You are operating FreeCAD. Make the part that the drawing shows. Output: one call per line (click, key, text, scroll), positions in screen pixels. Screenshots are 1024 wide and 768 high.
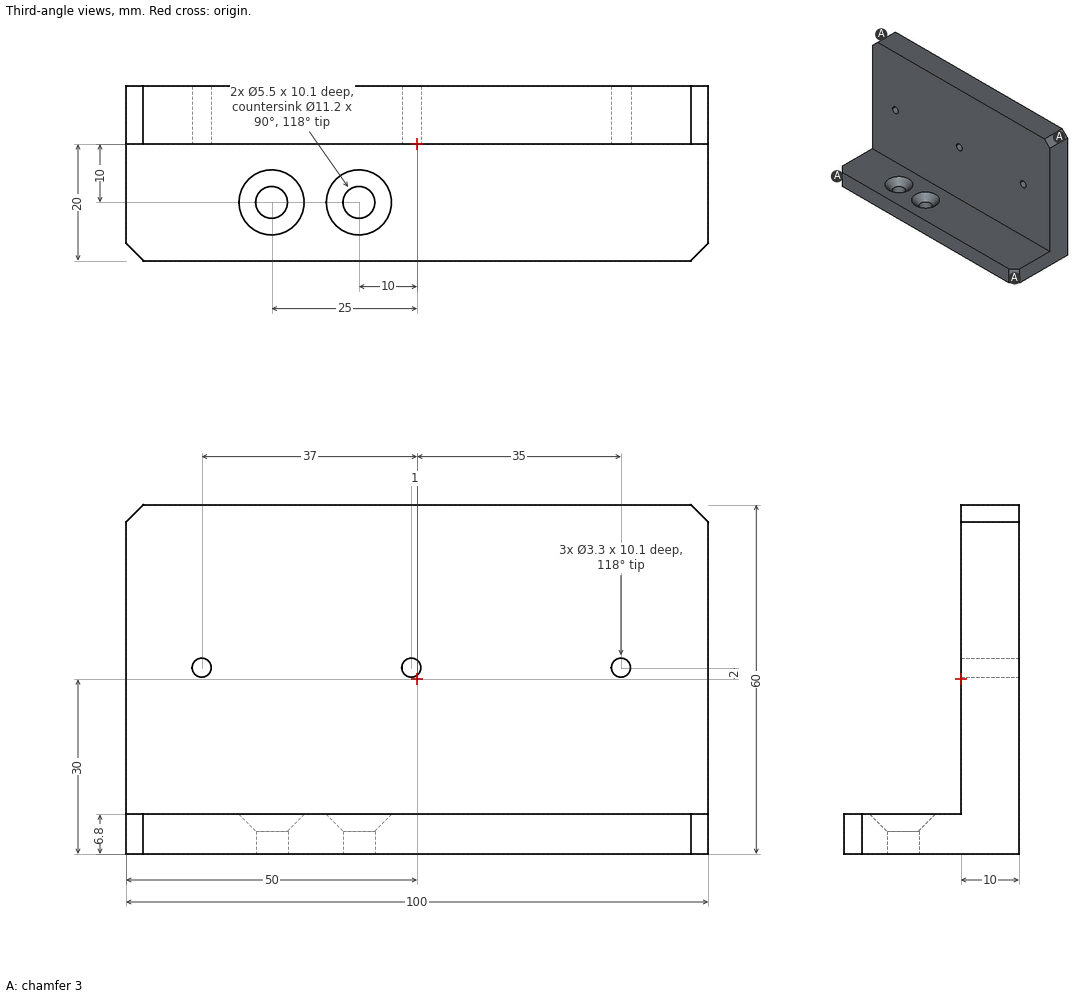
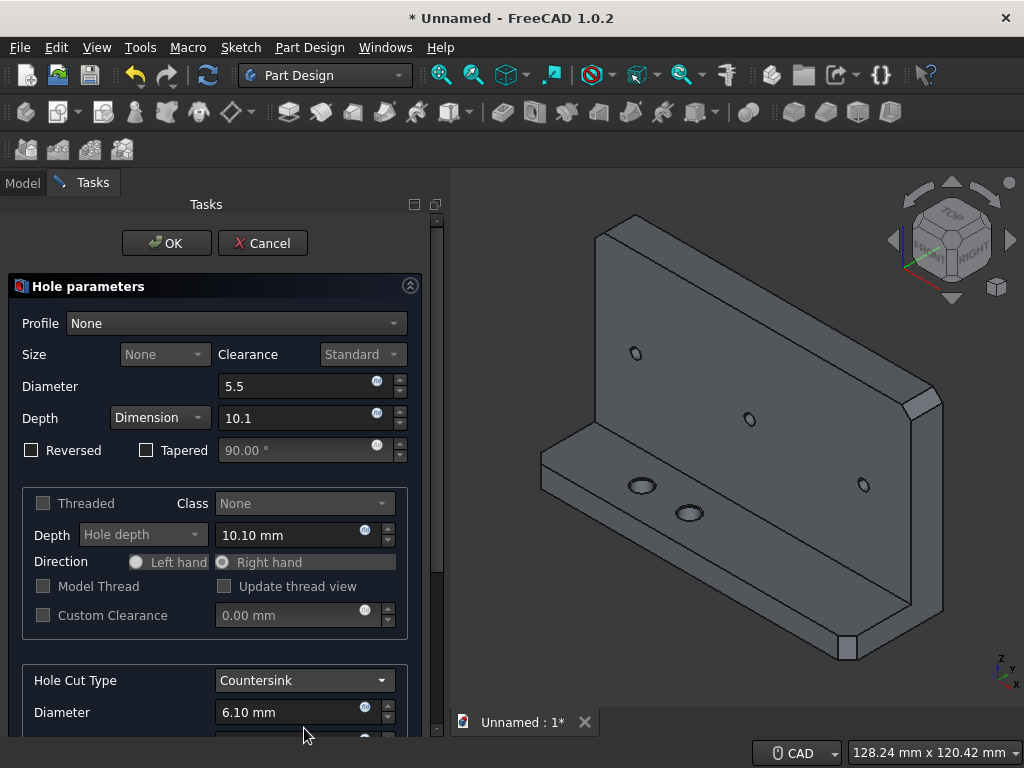
triple_click(298, 712)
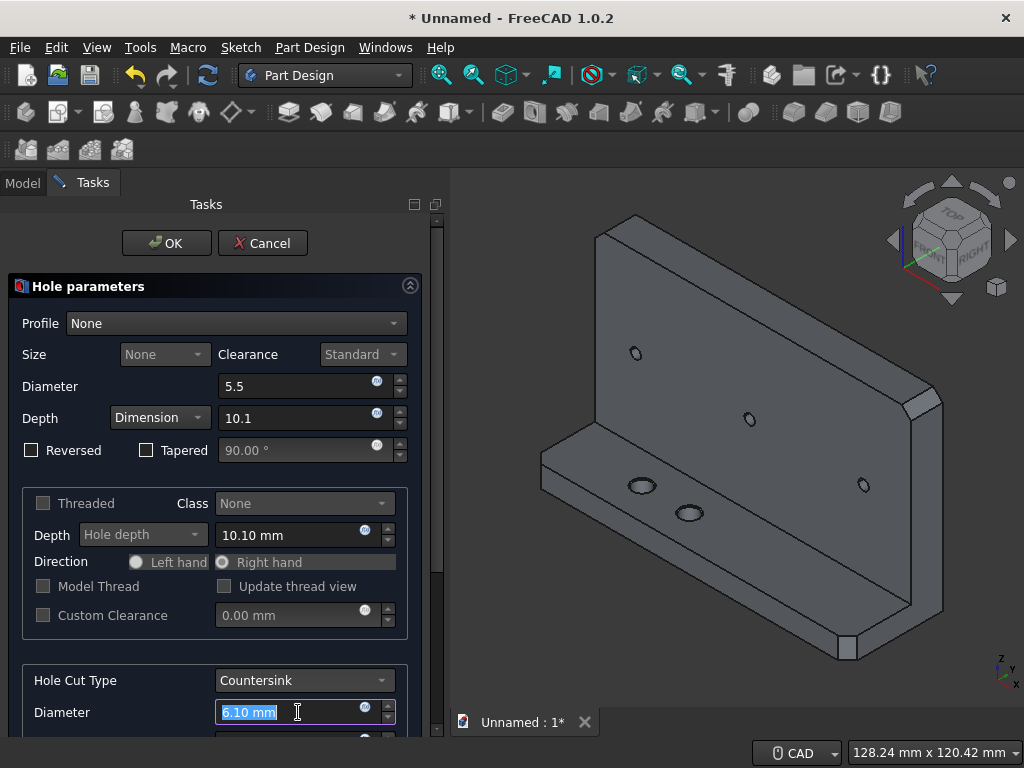
text(11.2)
key(Tab)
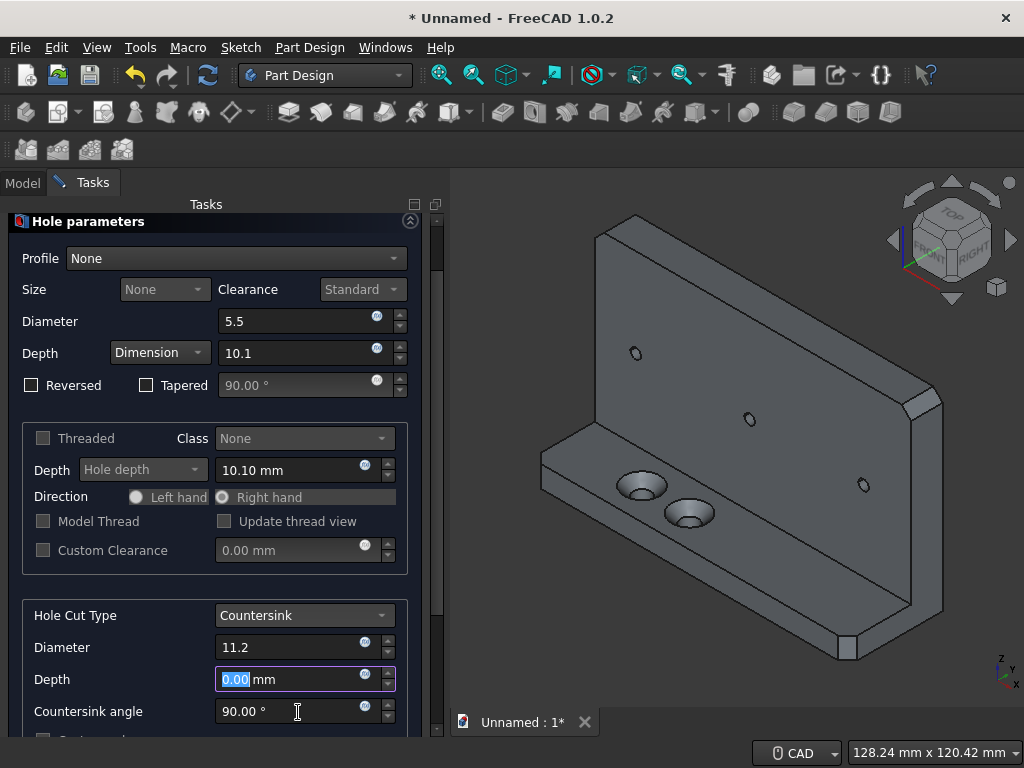
scroll(437, 475, up, 2)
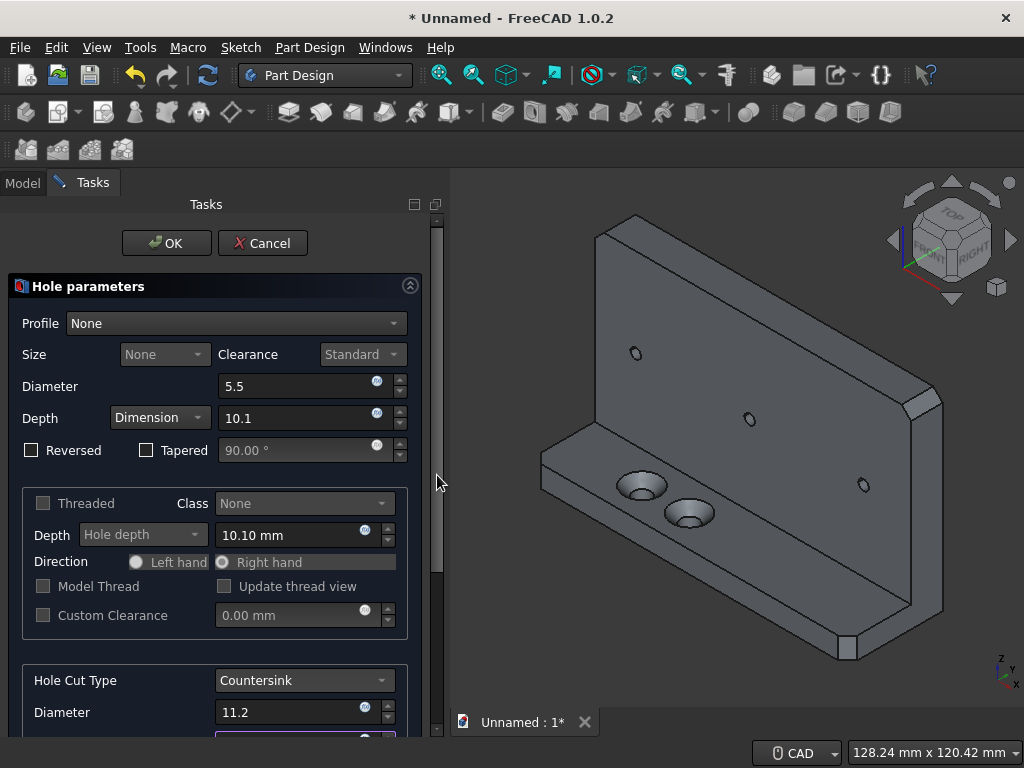
click(167, 243)